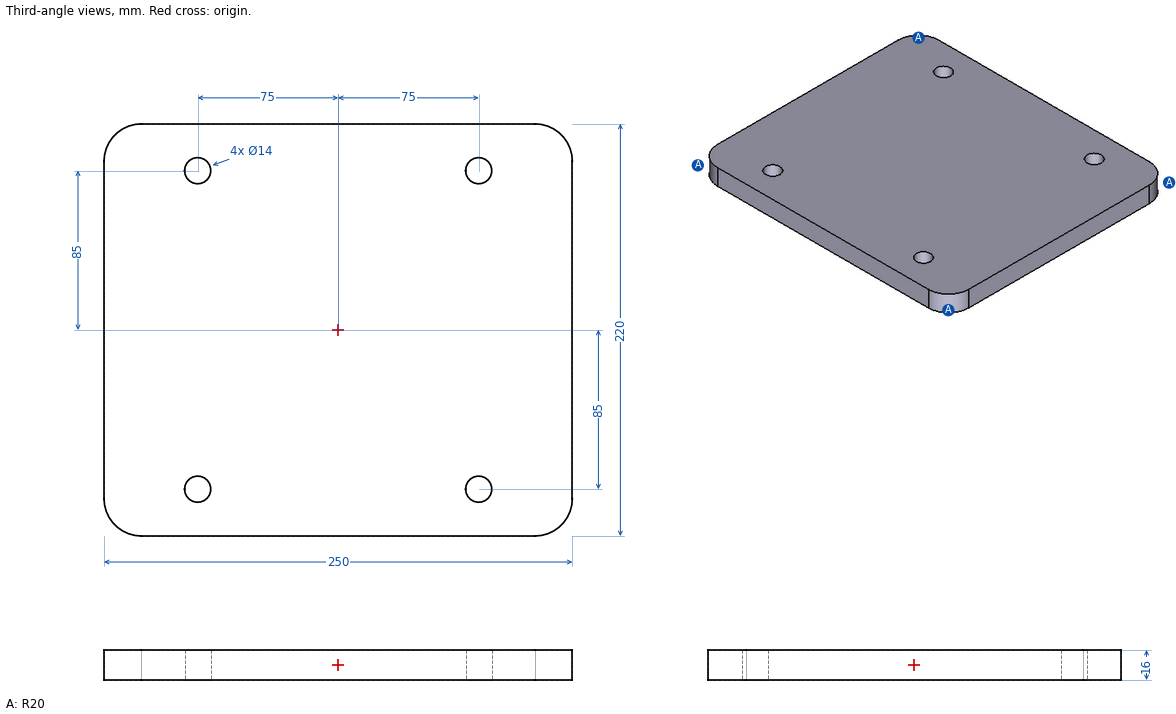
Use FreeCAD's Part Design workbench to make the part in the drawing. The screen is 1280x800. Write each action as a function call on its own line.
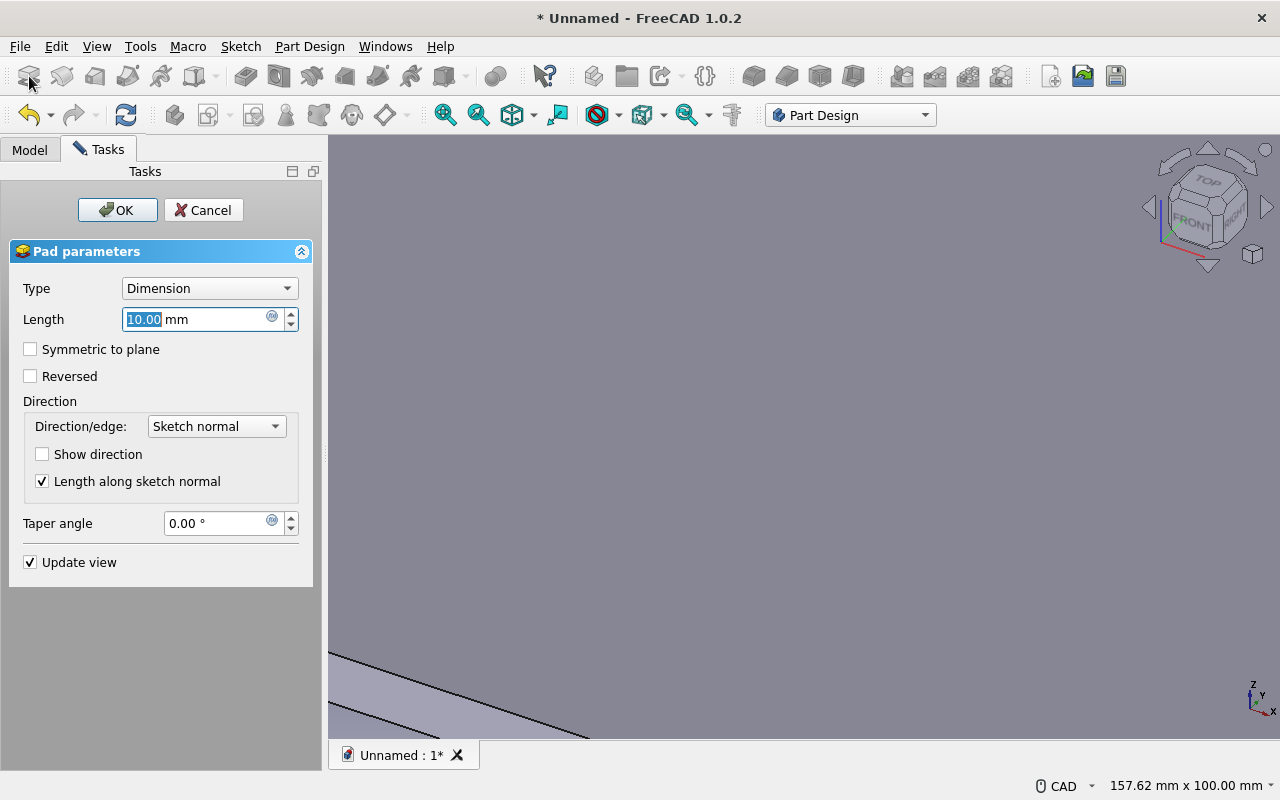
text(16)
key(Tab)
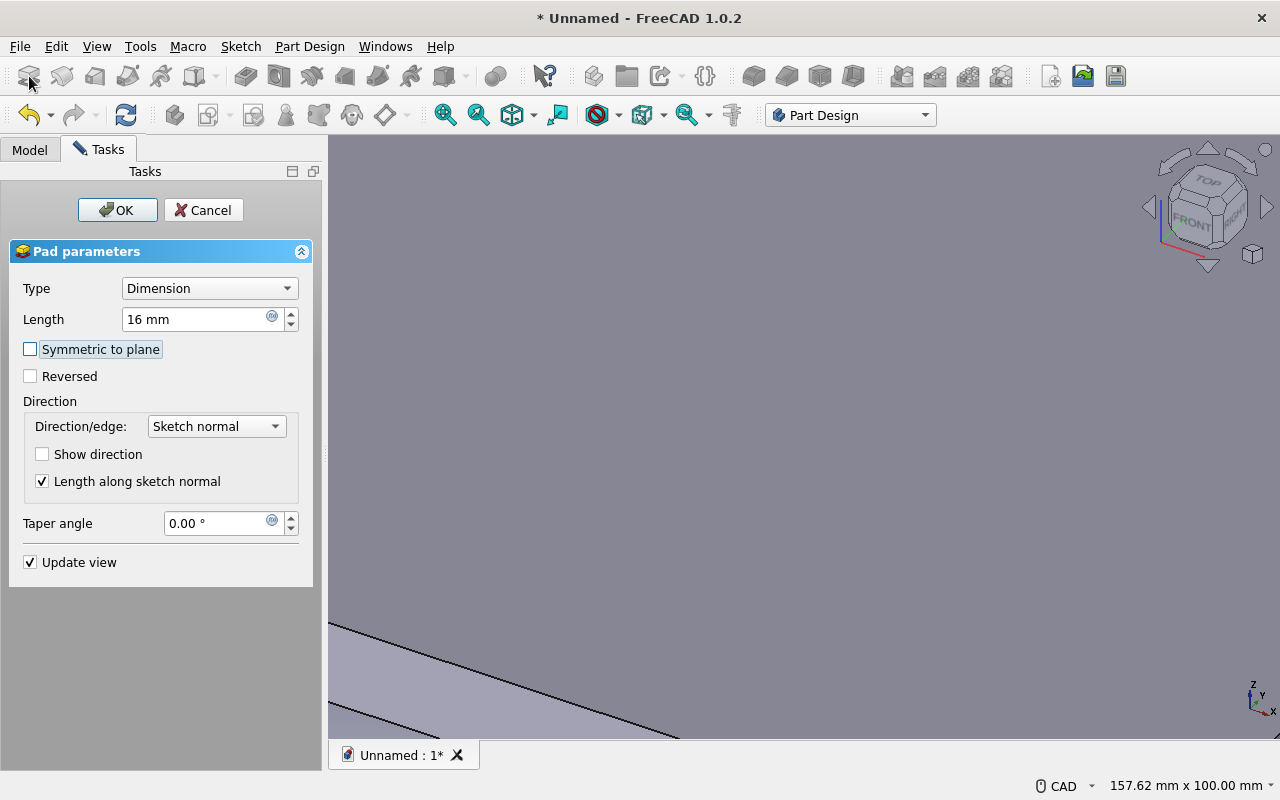
click(31, 349)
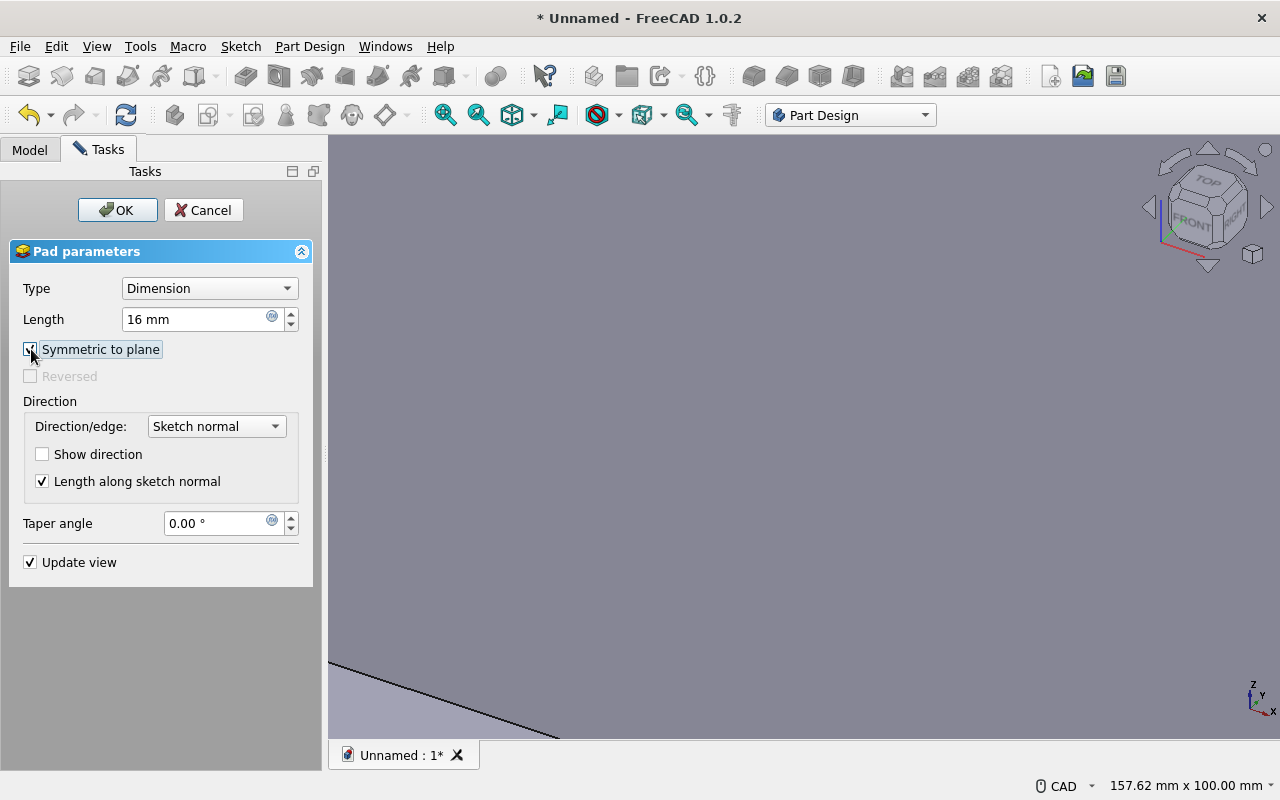
click(118, 210)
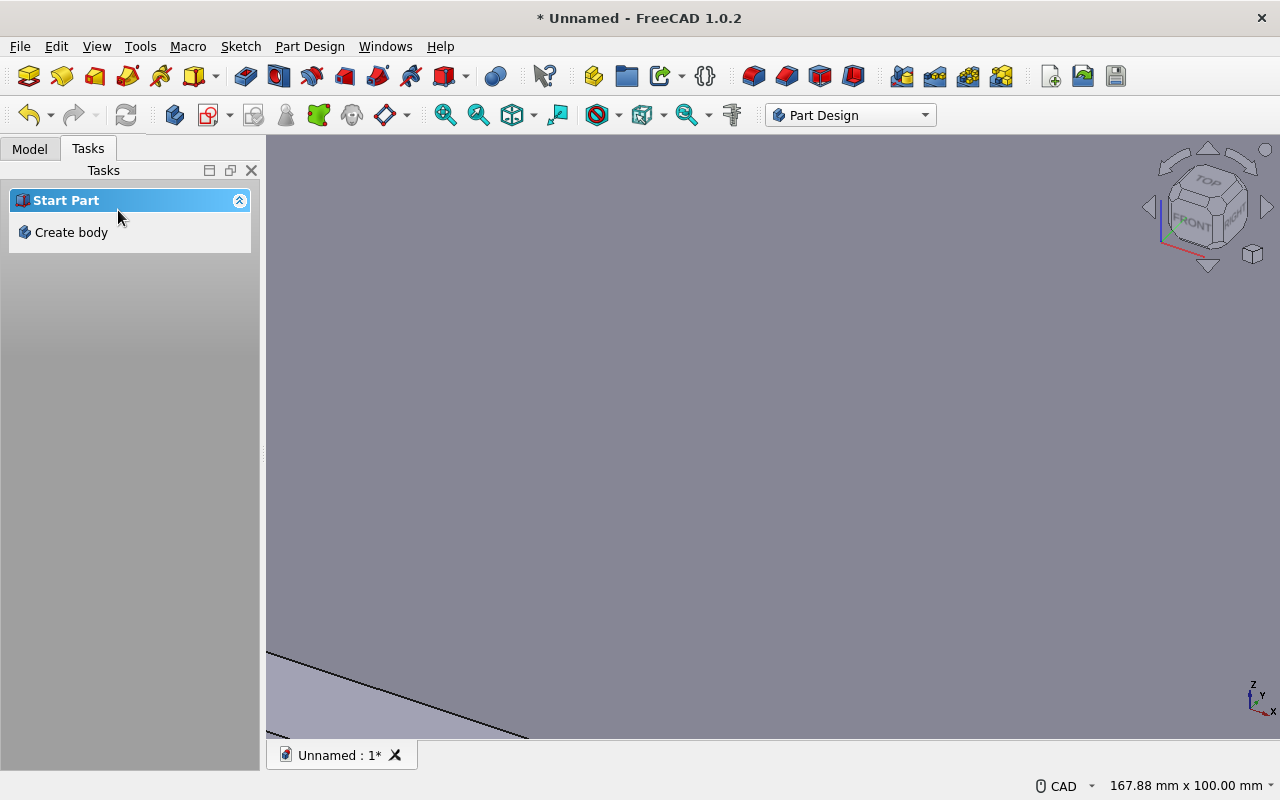
click(446, 116)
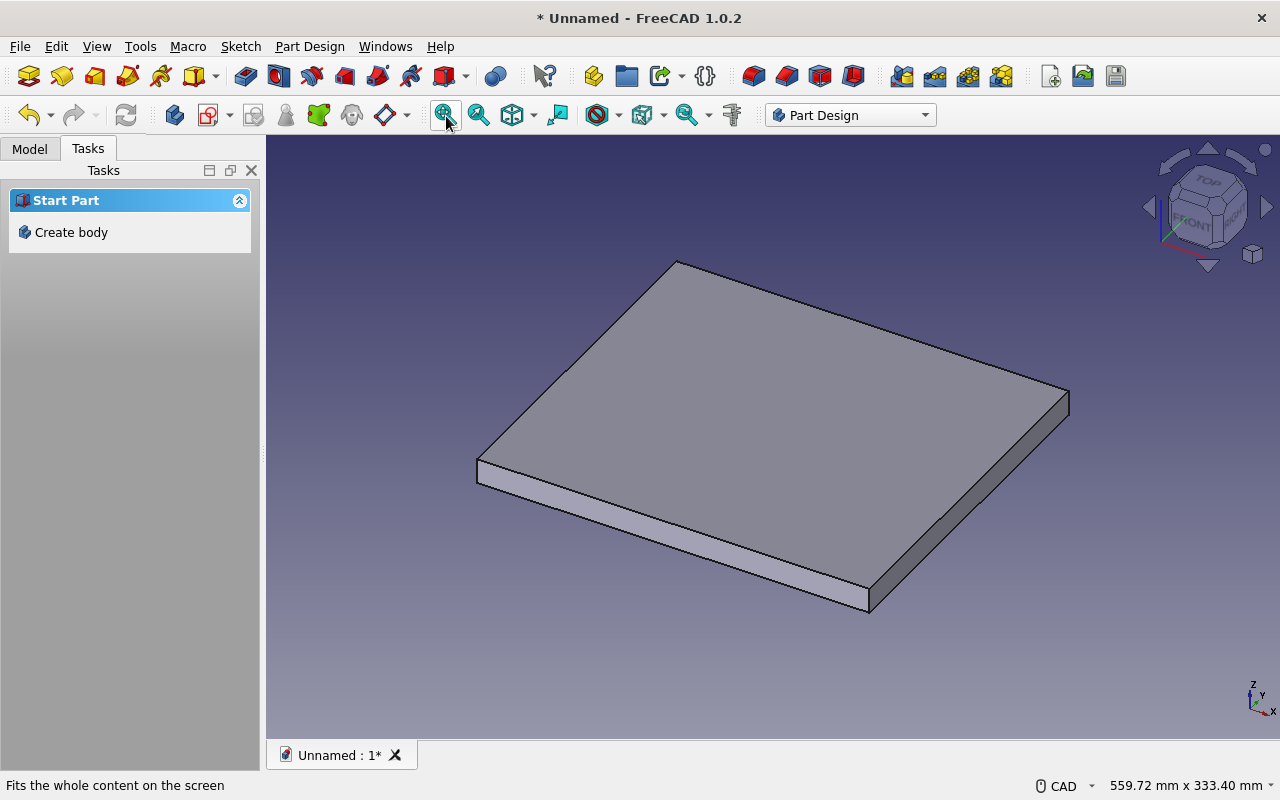
click(773, 424)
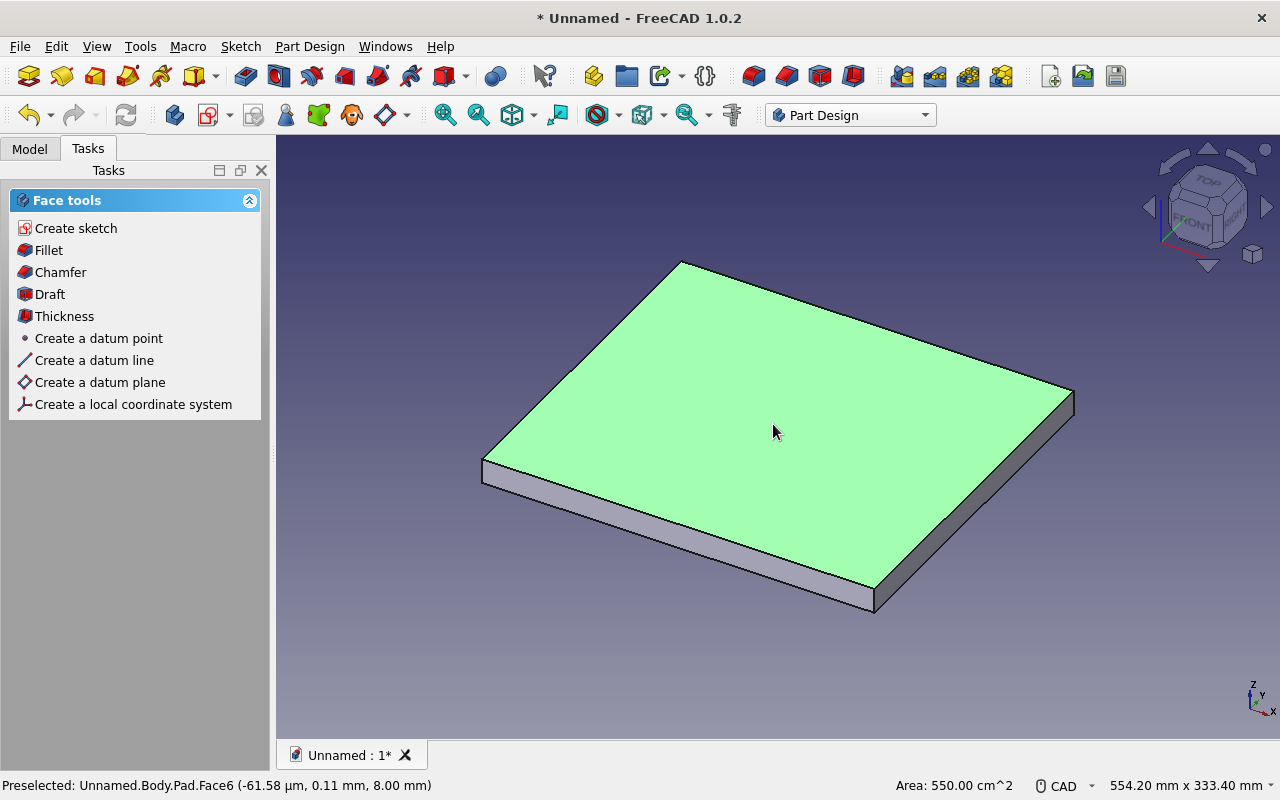
click(208, 116)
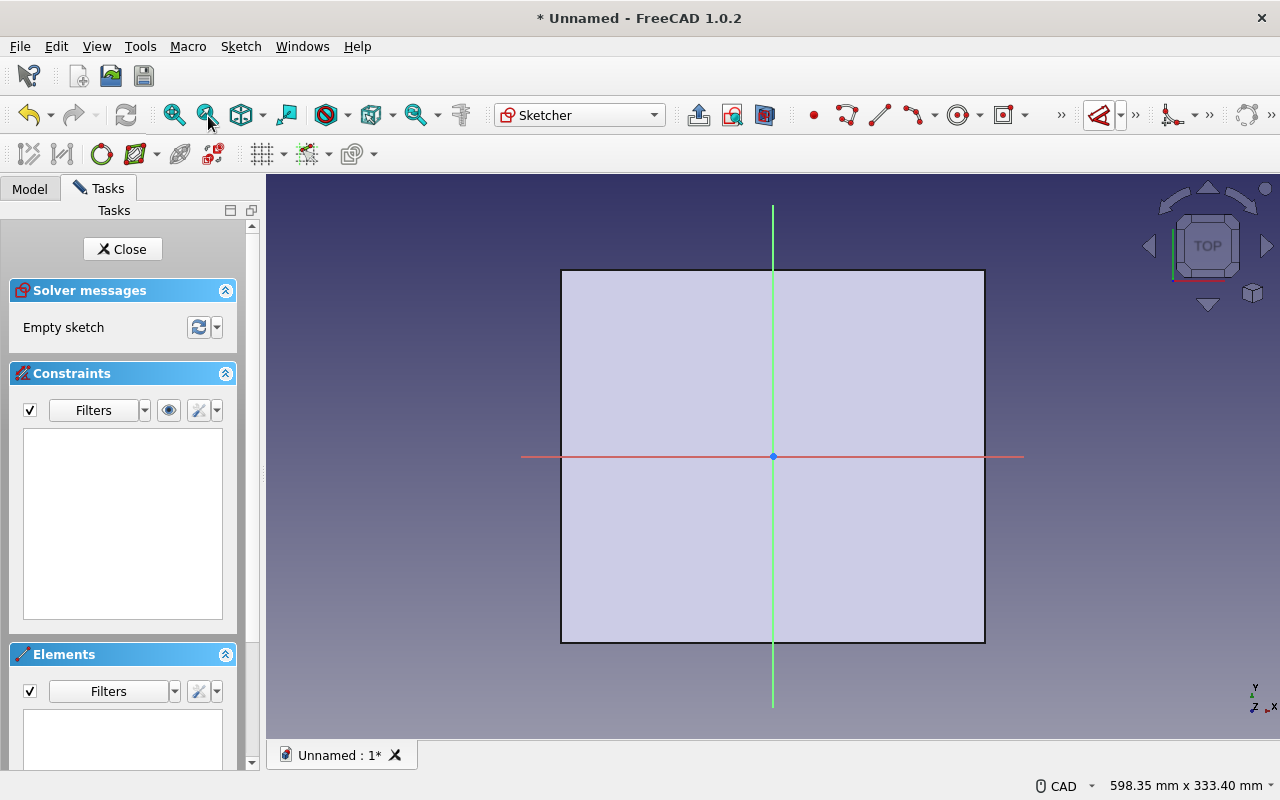
click(958, 116)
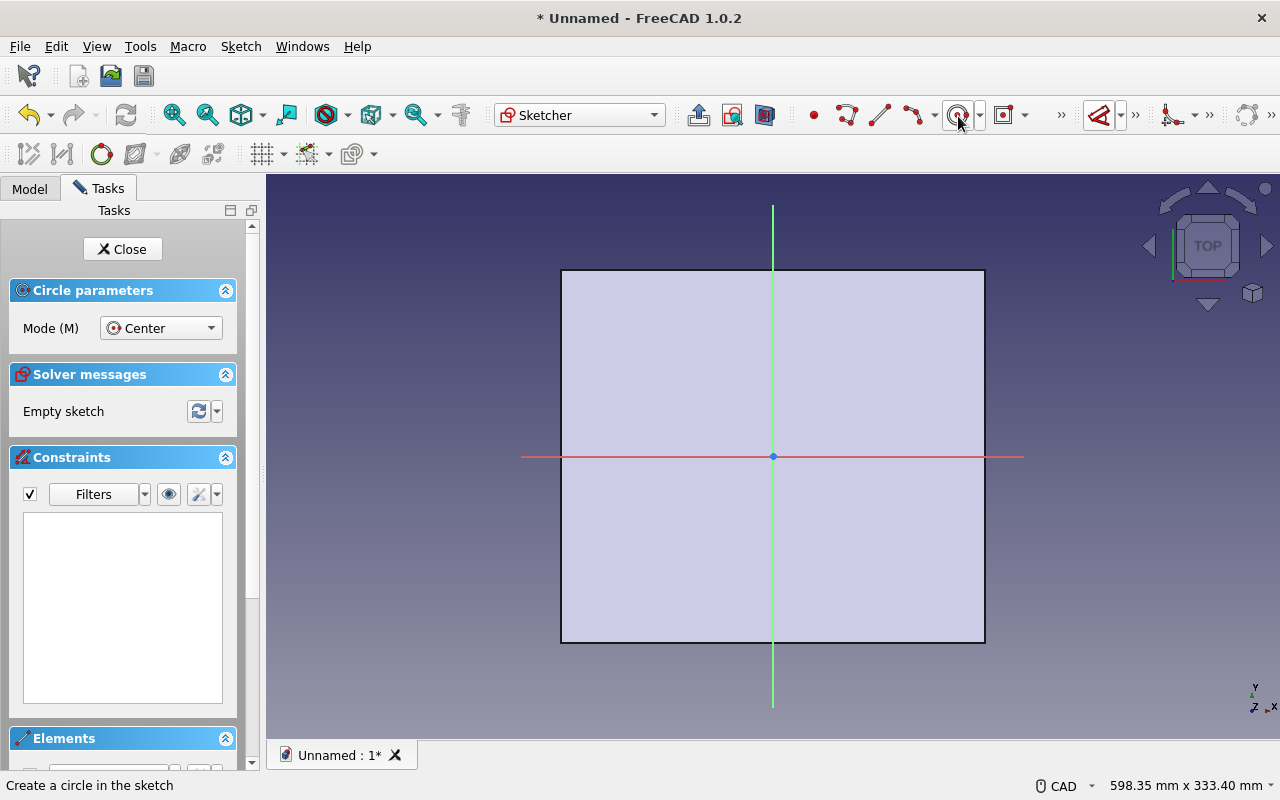
scroll(646, 312, up, 4)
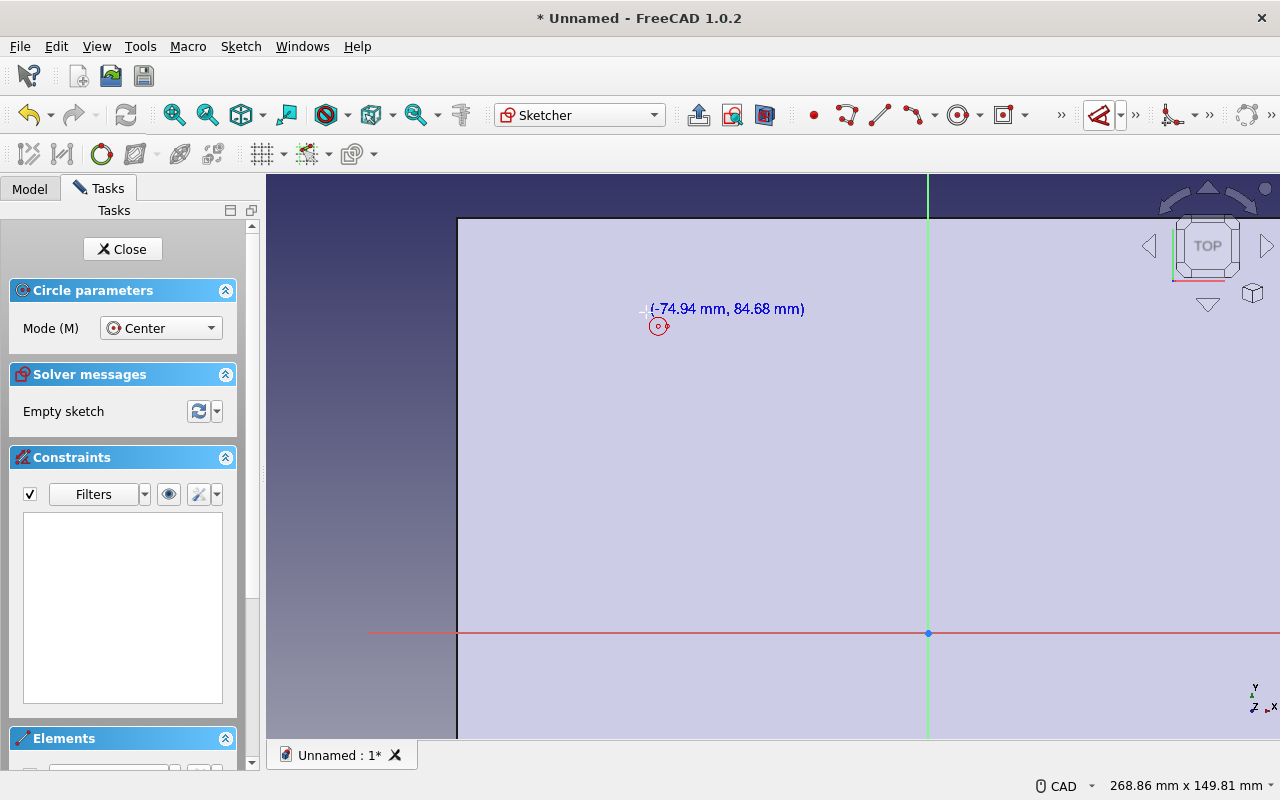
click(645, 313)
move(664, 294)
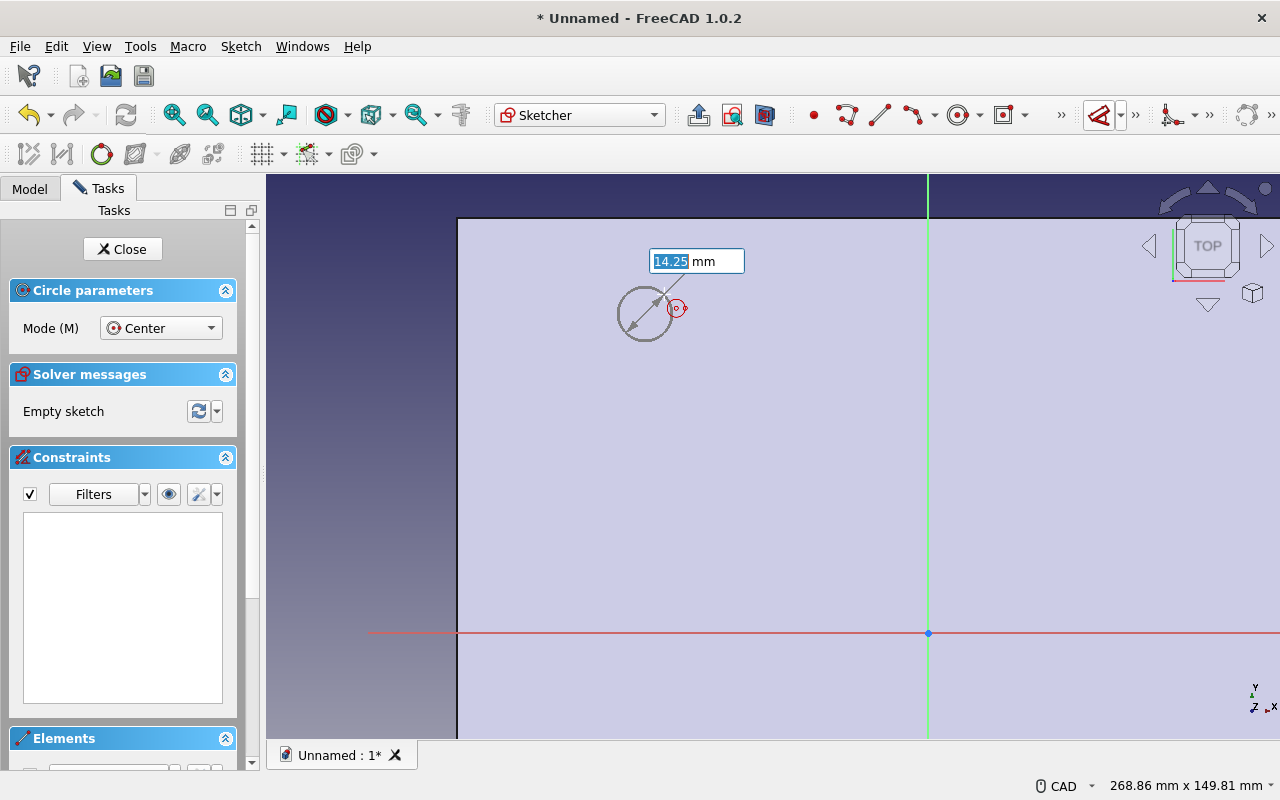
text(14)
key(Return)